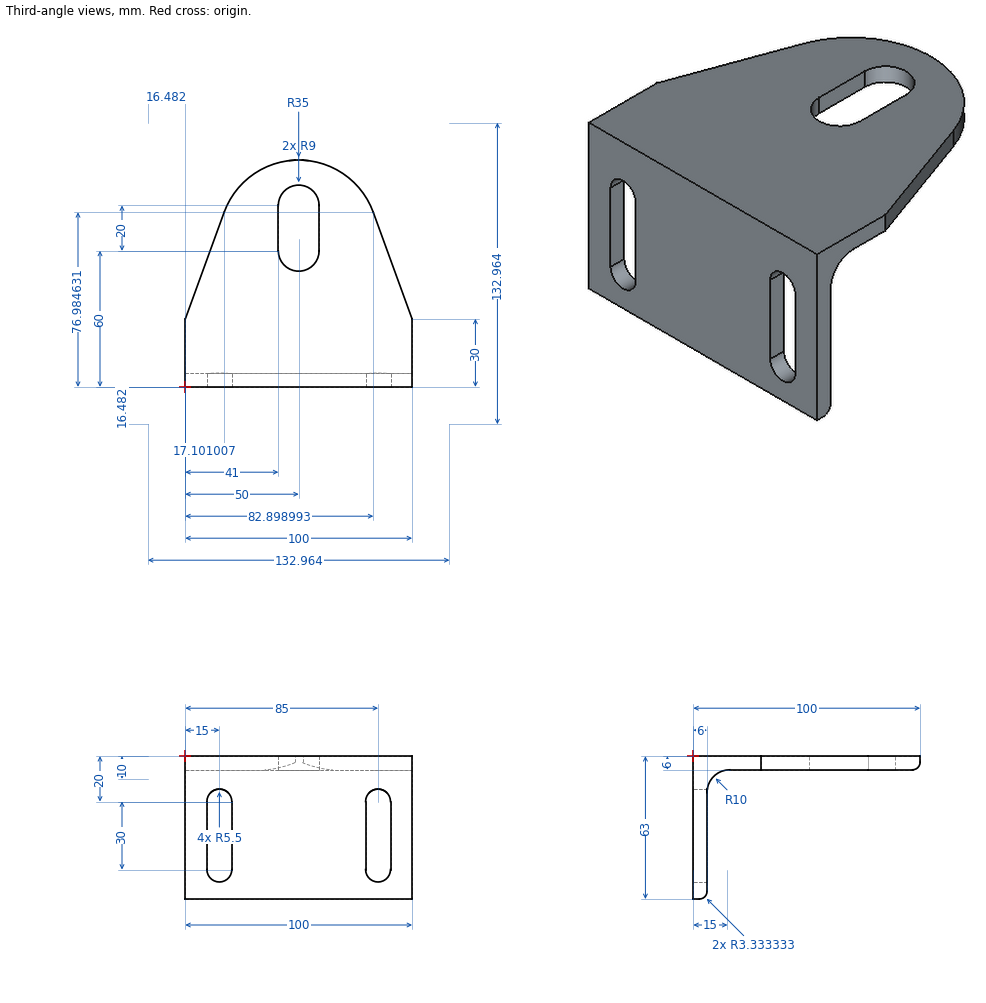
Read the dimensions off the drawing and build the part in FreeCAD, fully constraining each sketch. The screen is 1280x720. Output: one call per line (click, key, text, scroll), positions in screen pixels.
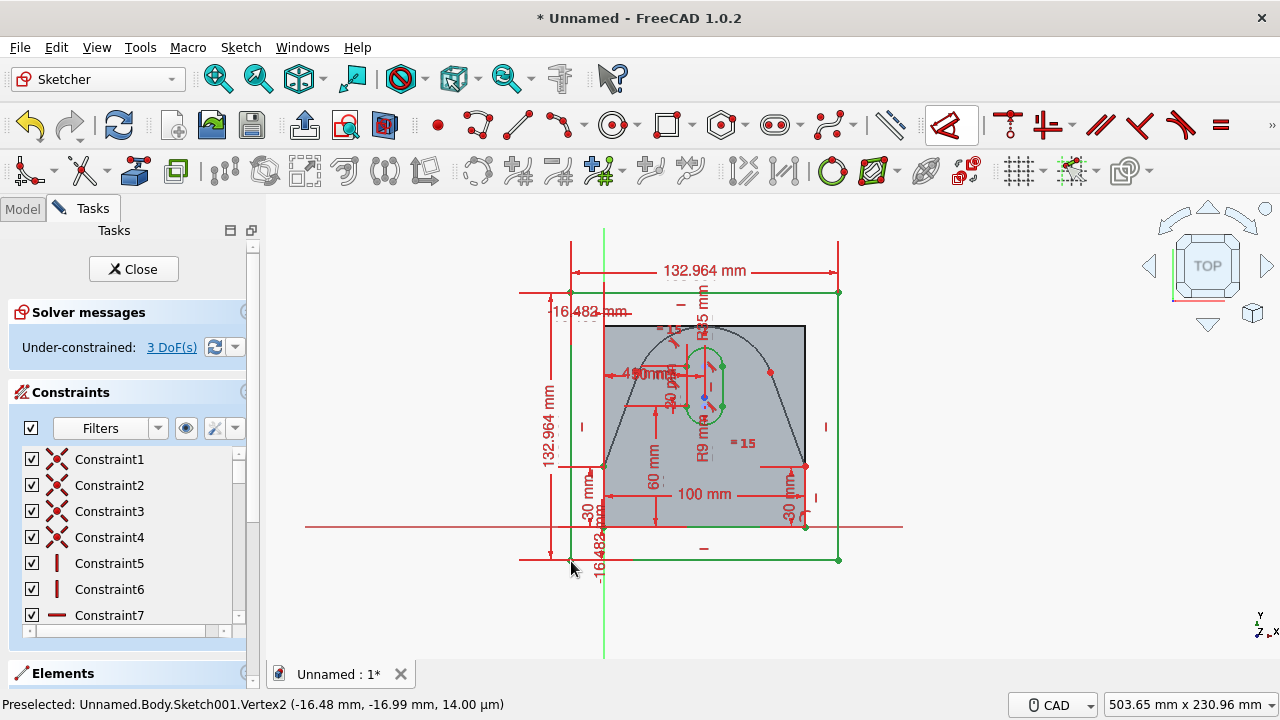
click(771, 373)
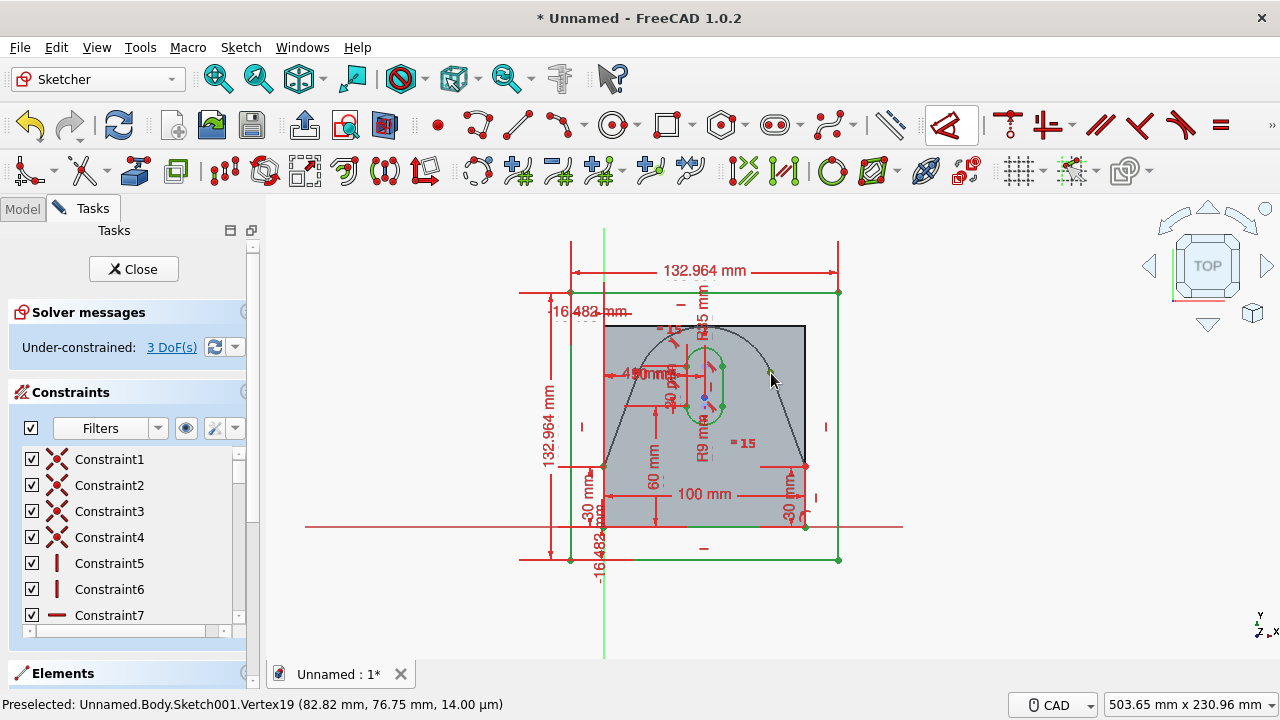
click(972, 126)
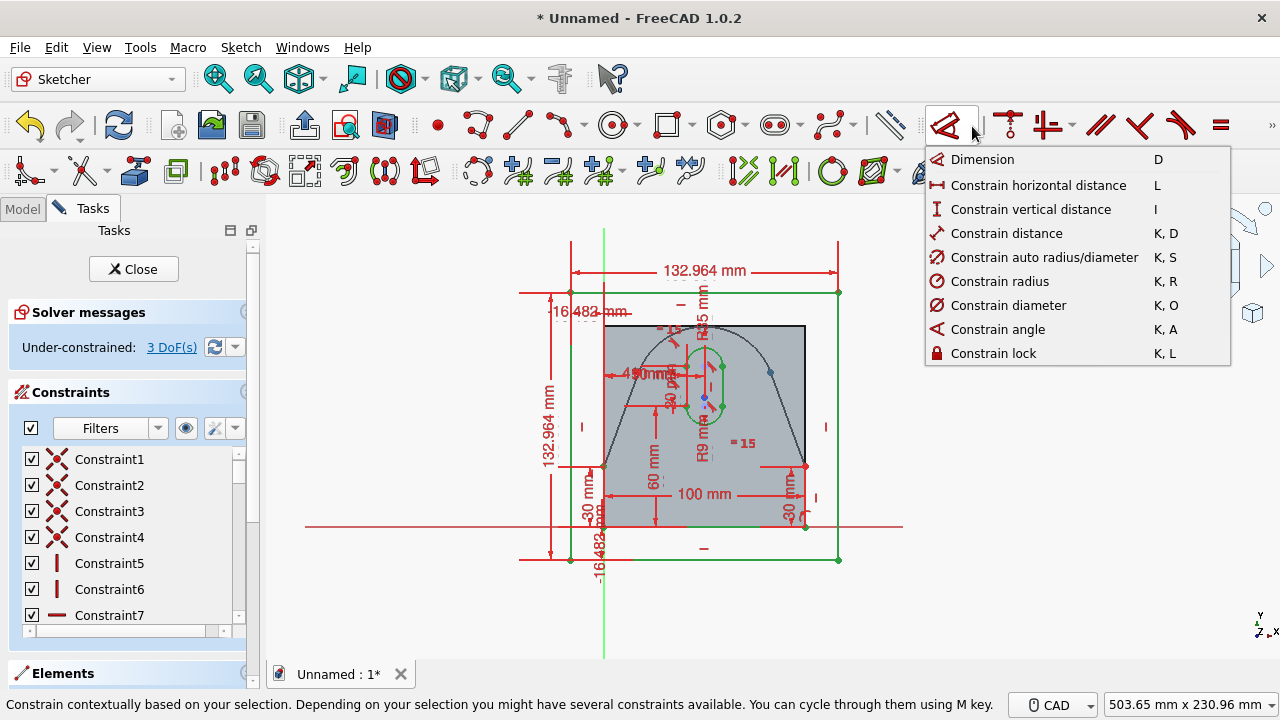
click(1078, 185)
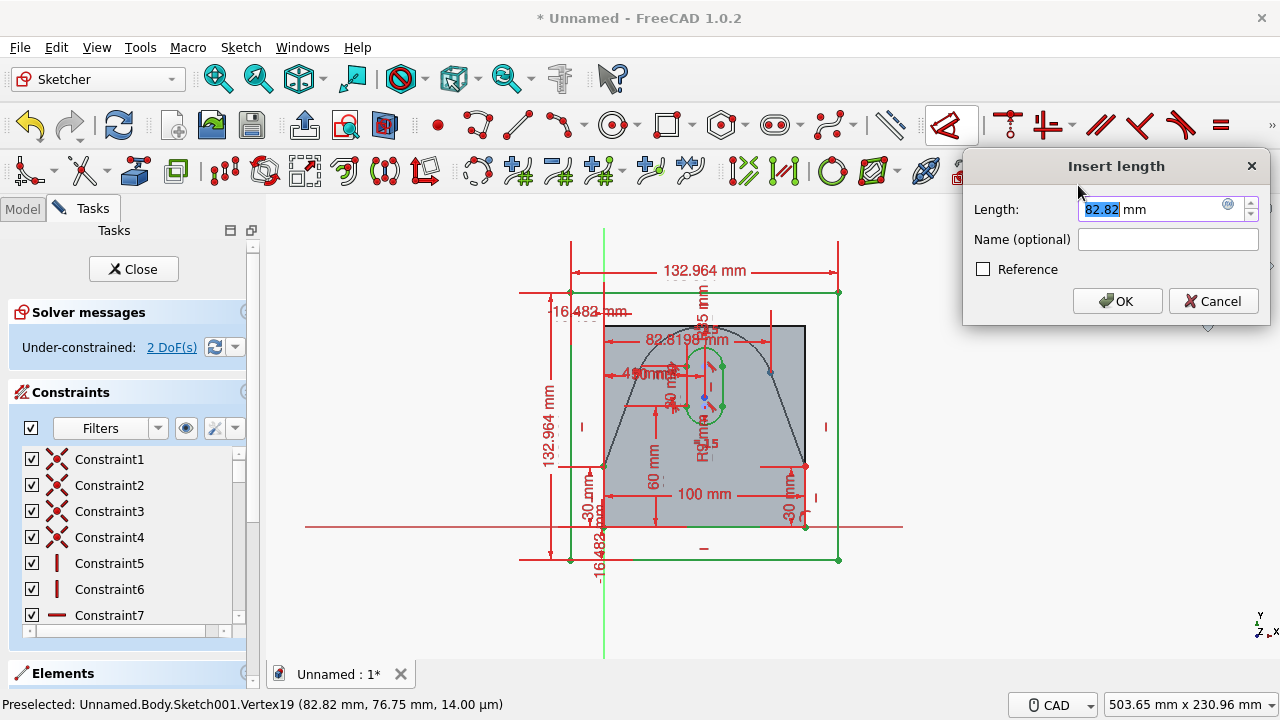
text(82.898993)
key(Return)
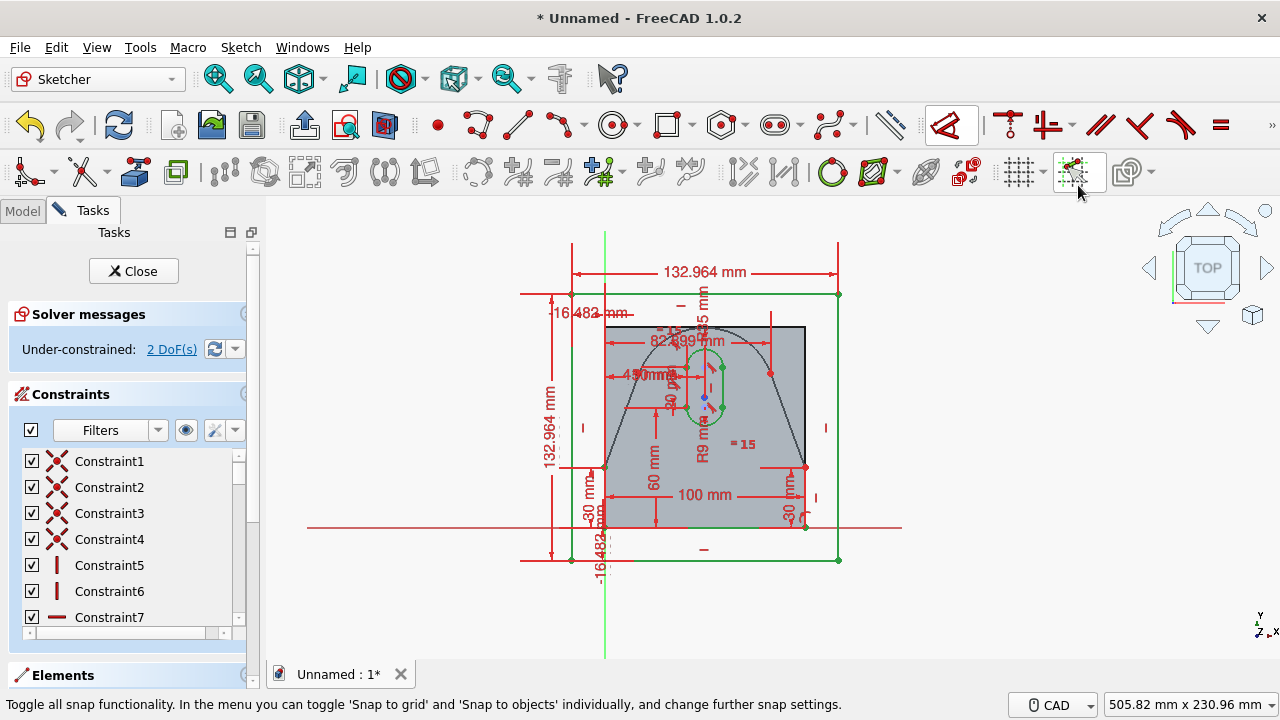
click(771, 374)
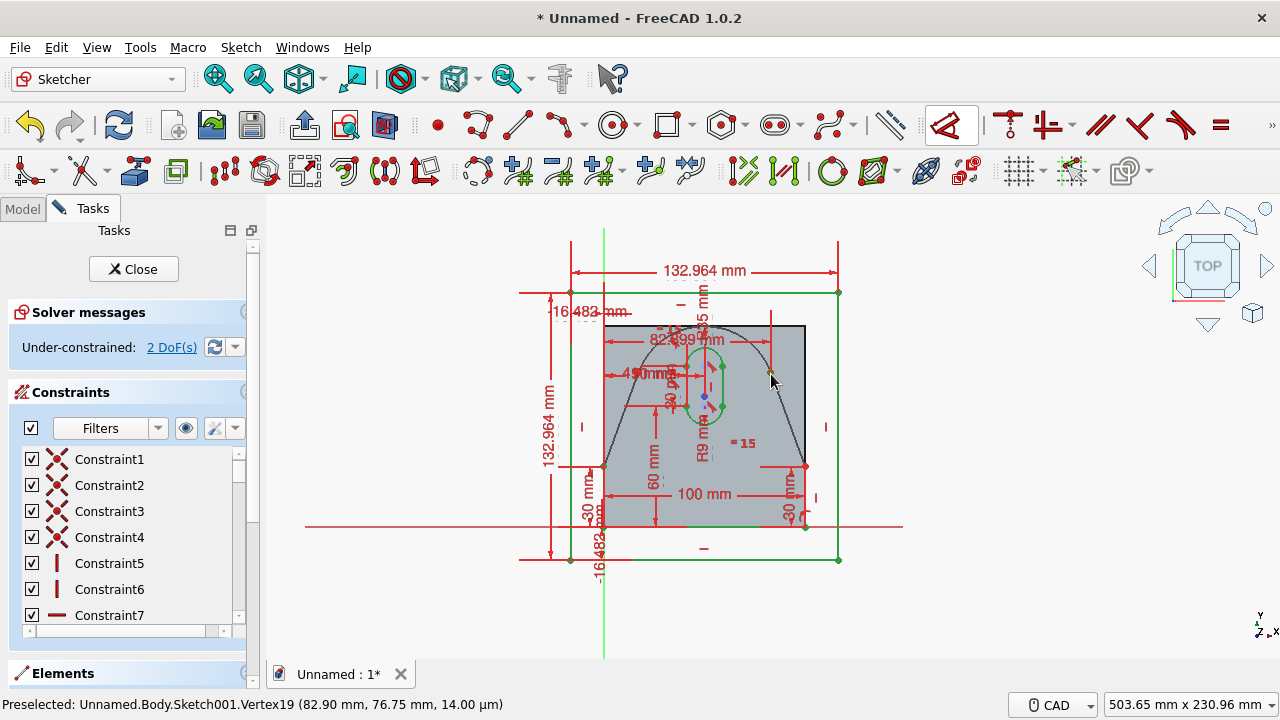
click(972, 126)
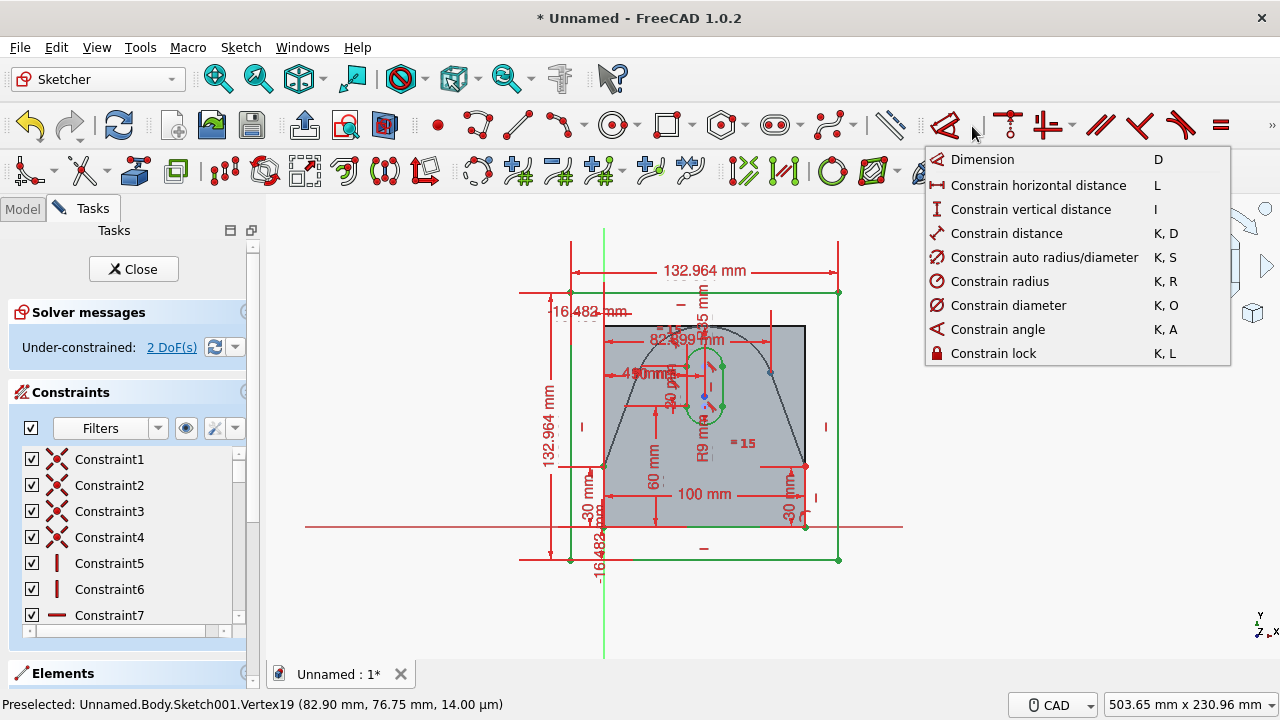
click(1078, 209)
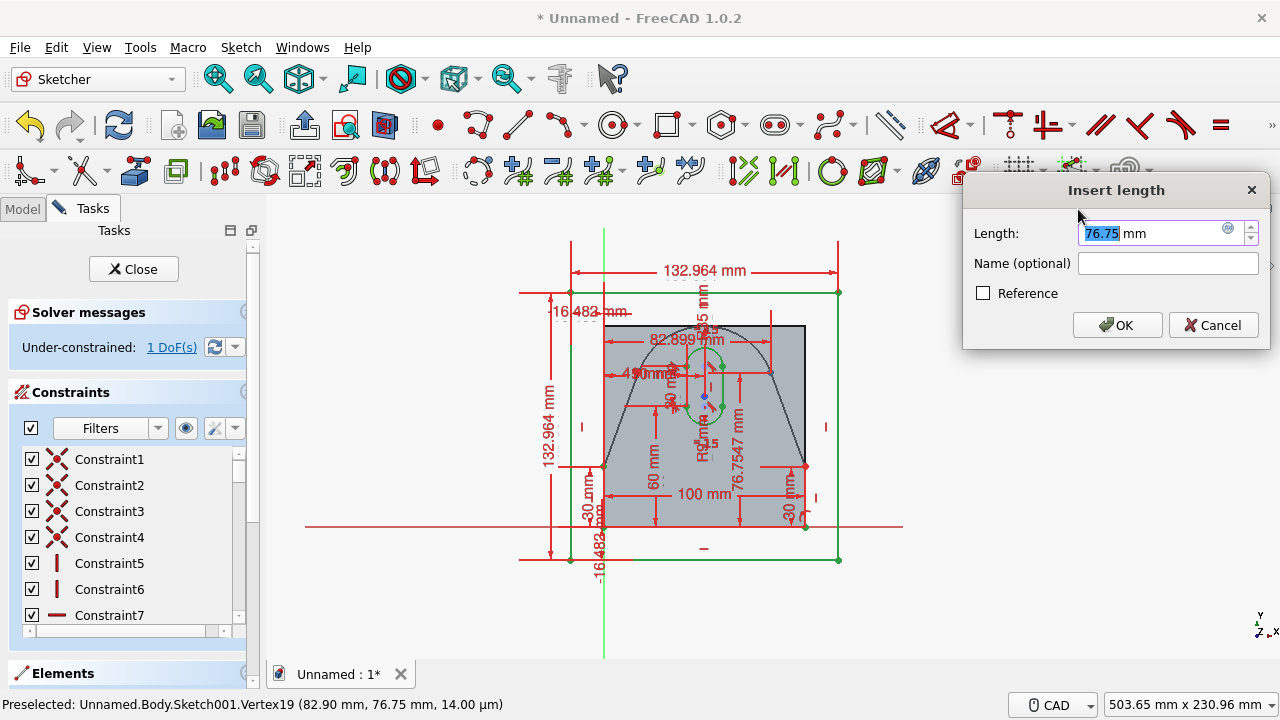
text(76.984631)
key(Return)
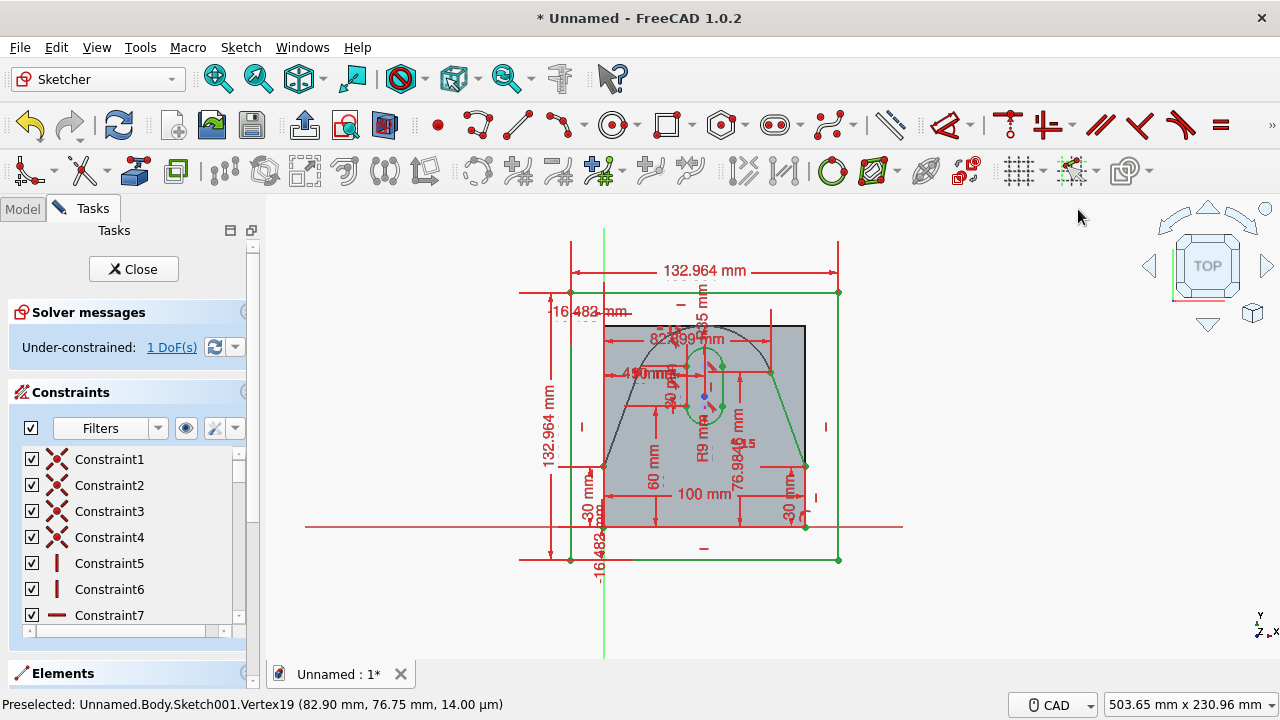
click(638, 373)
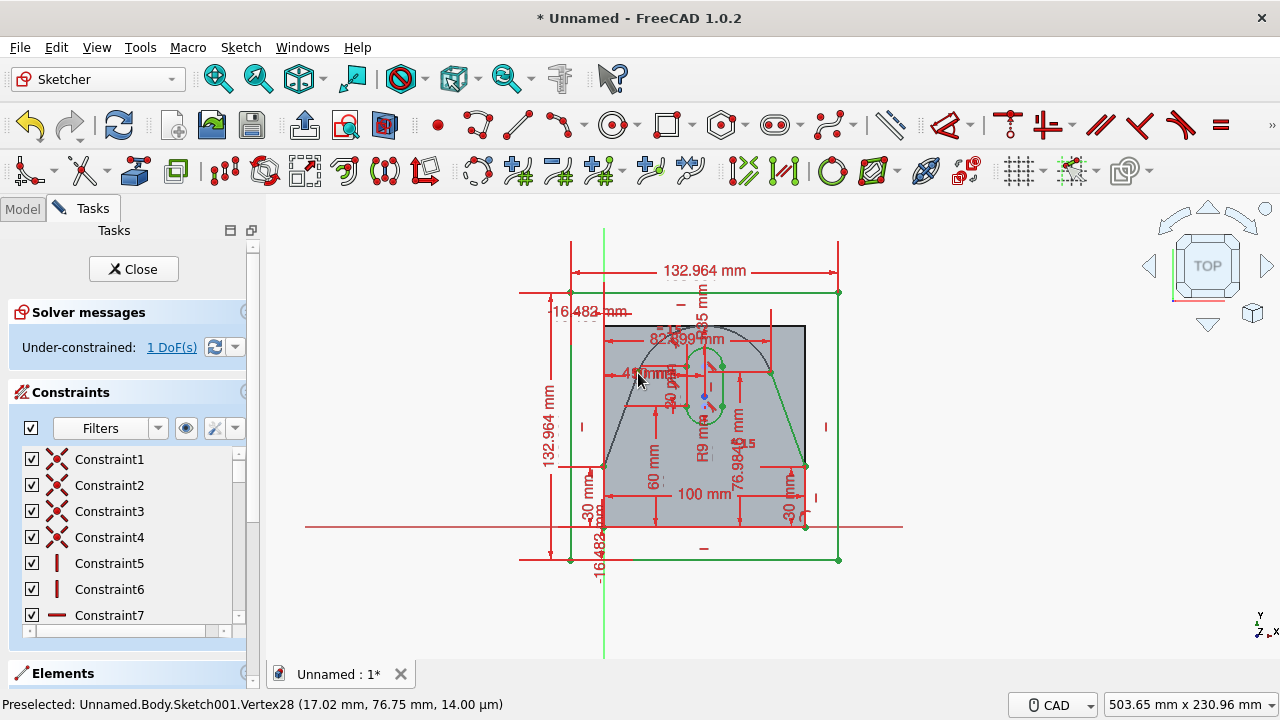
key(l)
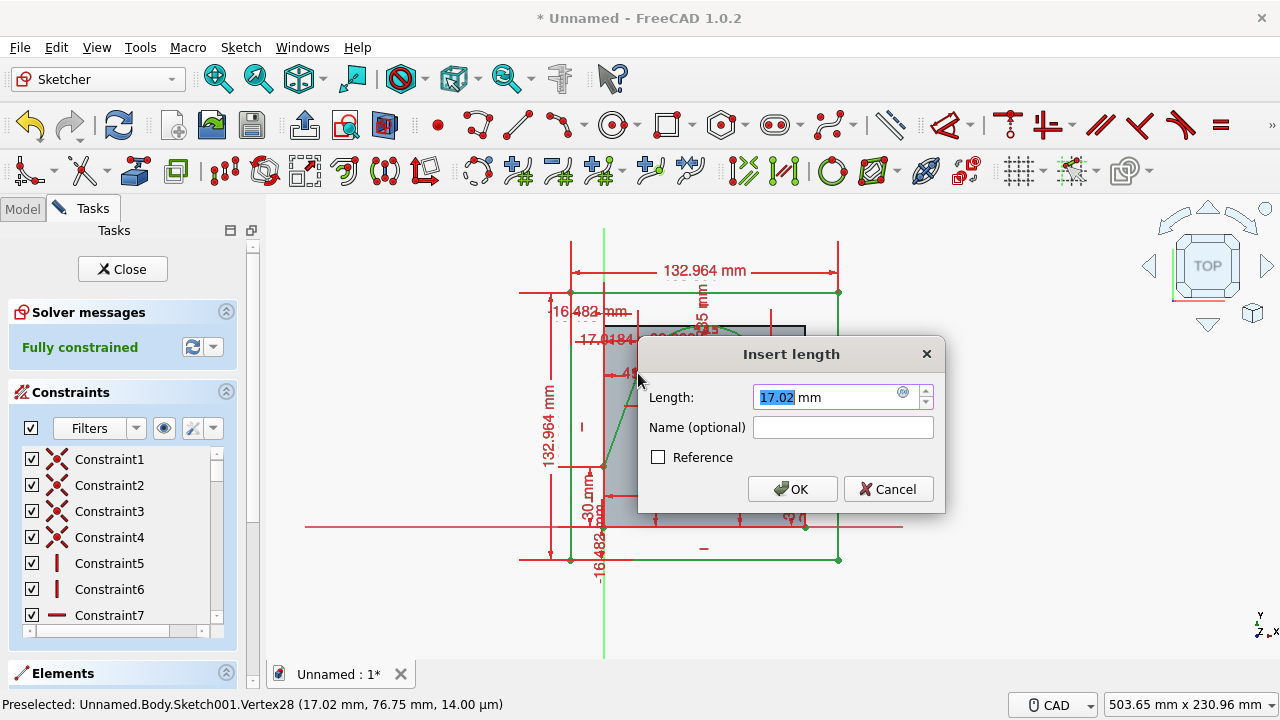
text(17.101007)
key(Return)